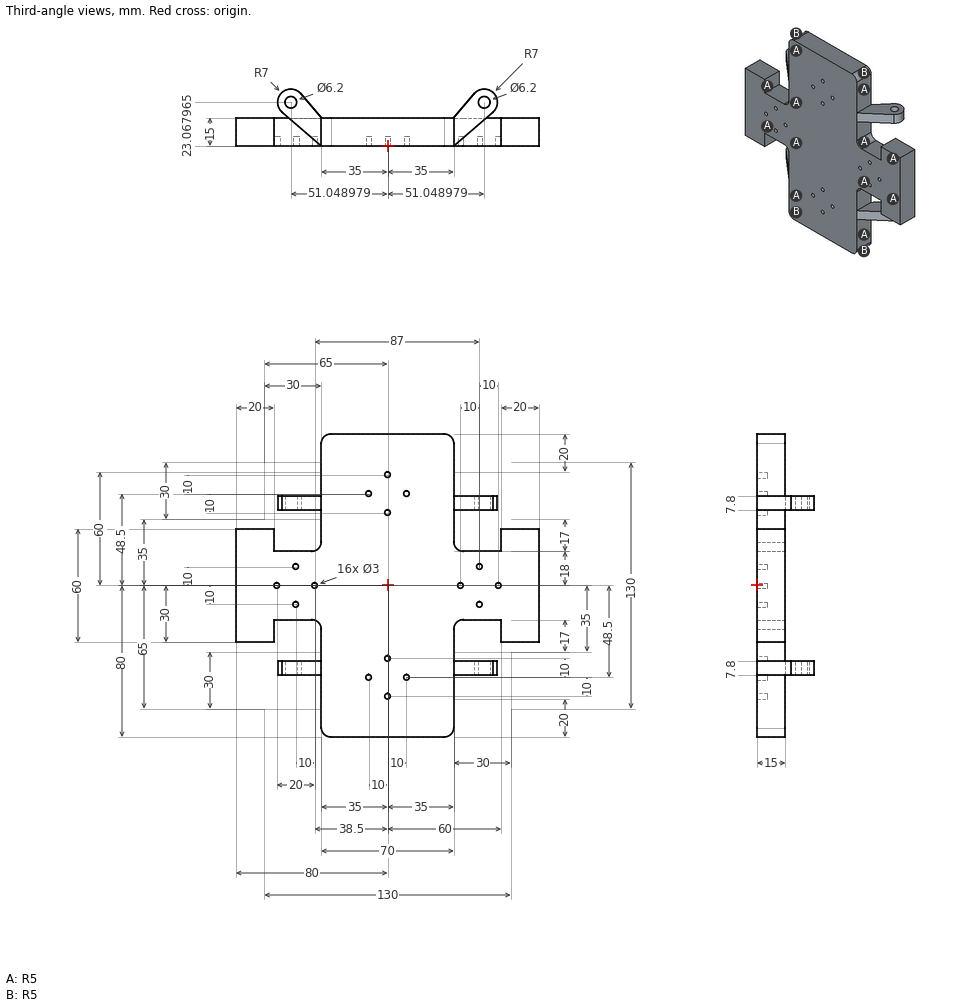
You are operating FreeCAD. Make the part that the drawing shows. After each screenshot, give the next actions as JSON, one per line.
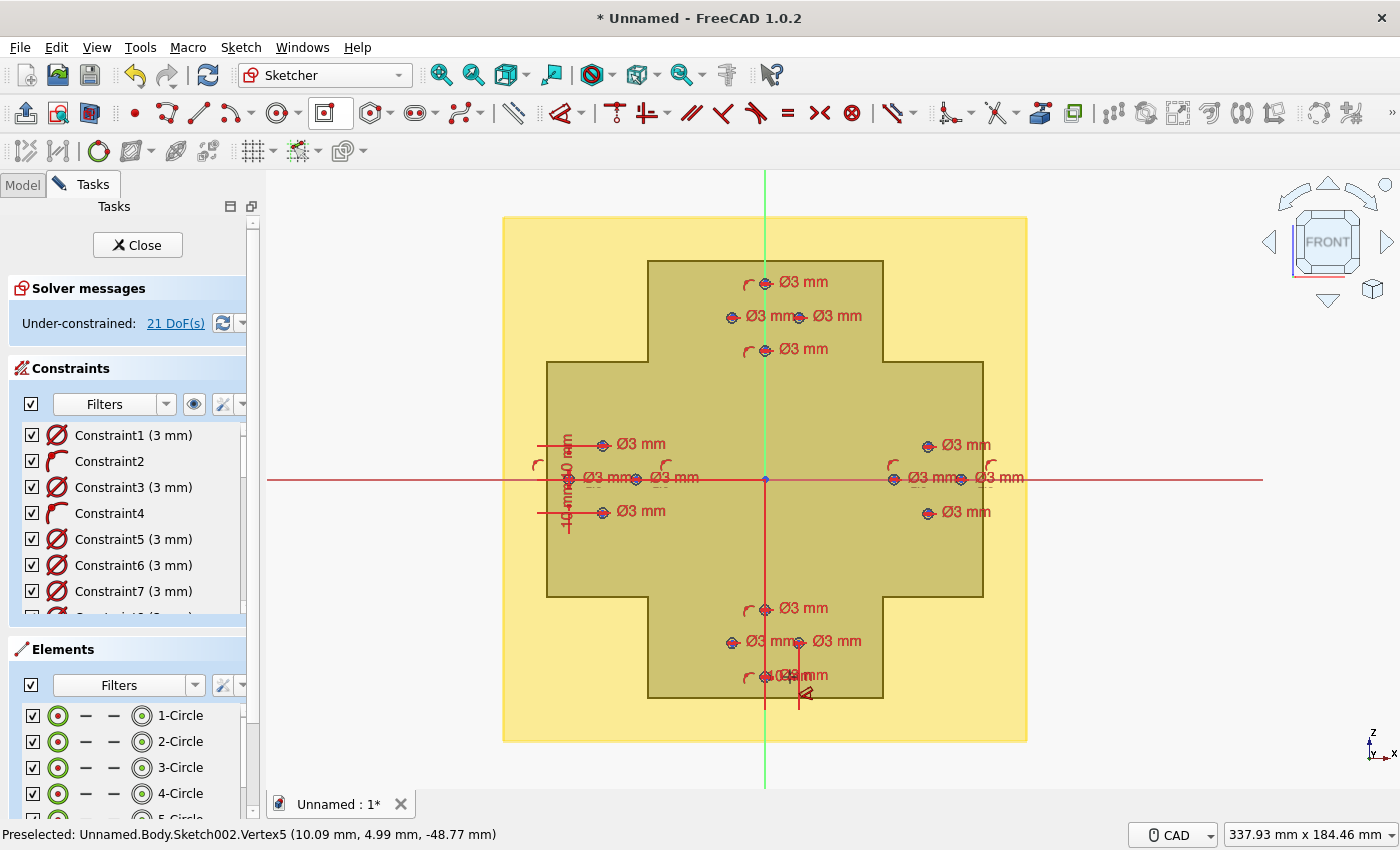
{"action": "left_click", "coordinate": [732, 643]}
{"action": "left_click", "coordinate": [749, 446]}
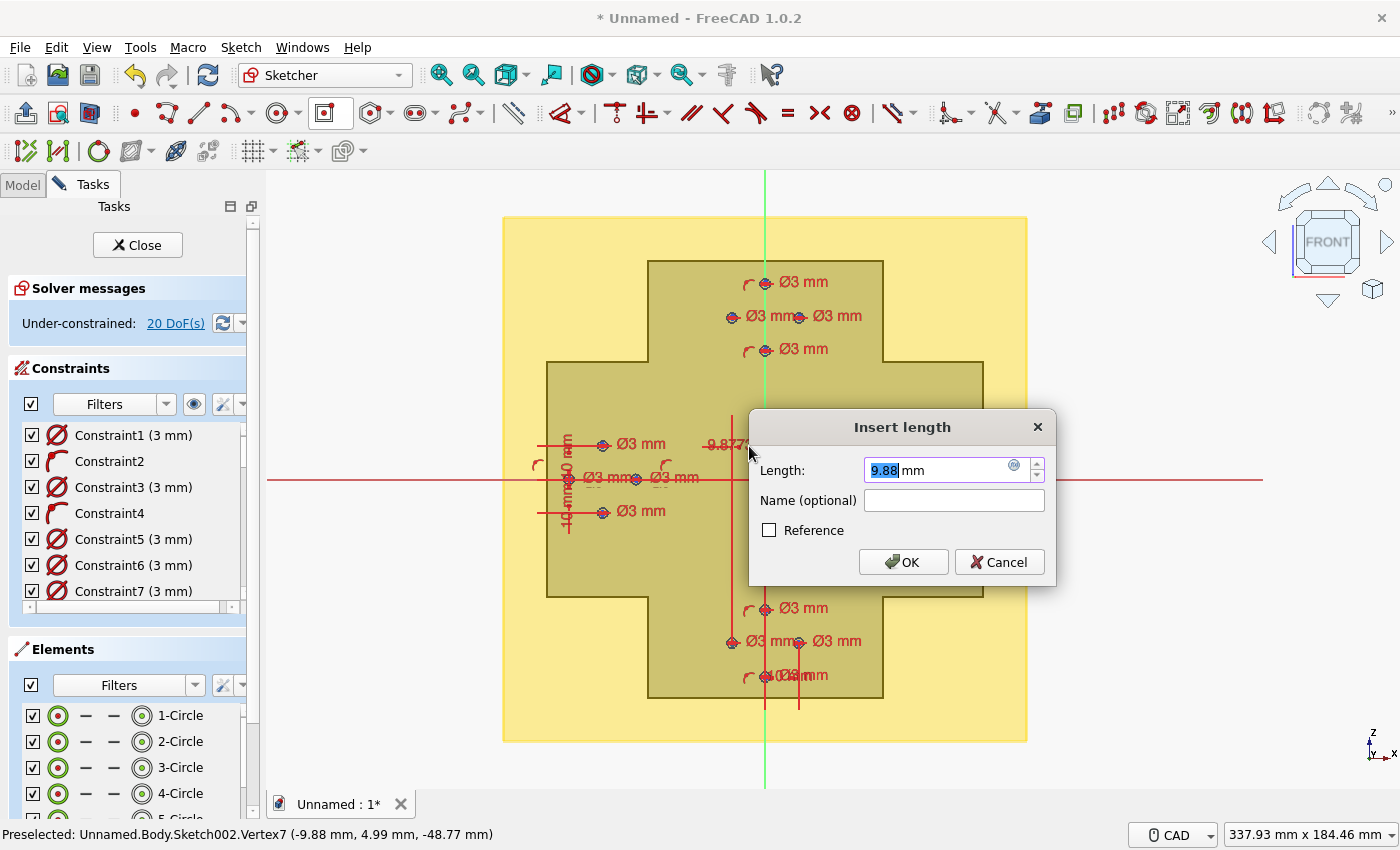
{"action": "type", "text": "10"}
{"action": "key", "text": "Return"}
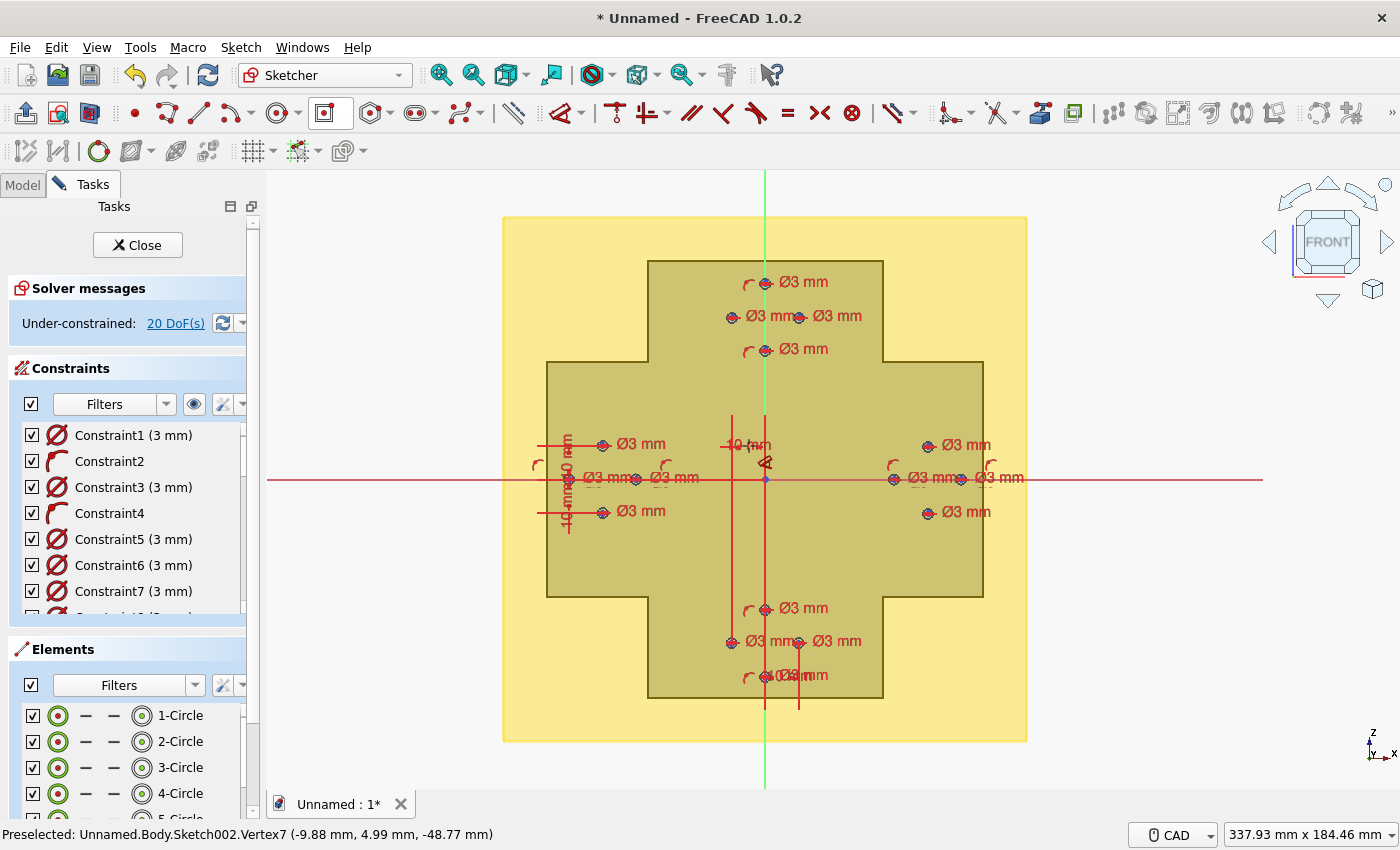
{"action": "left_click", "coordinate": [928, 447]}
{"action": "left_click", "coordinate": [962, 456]}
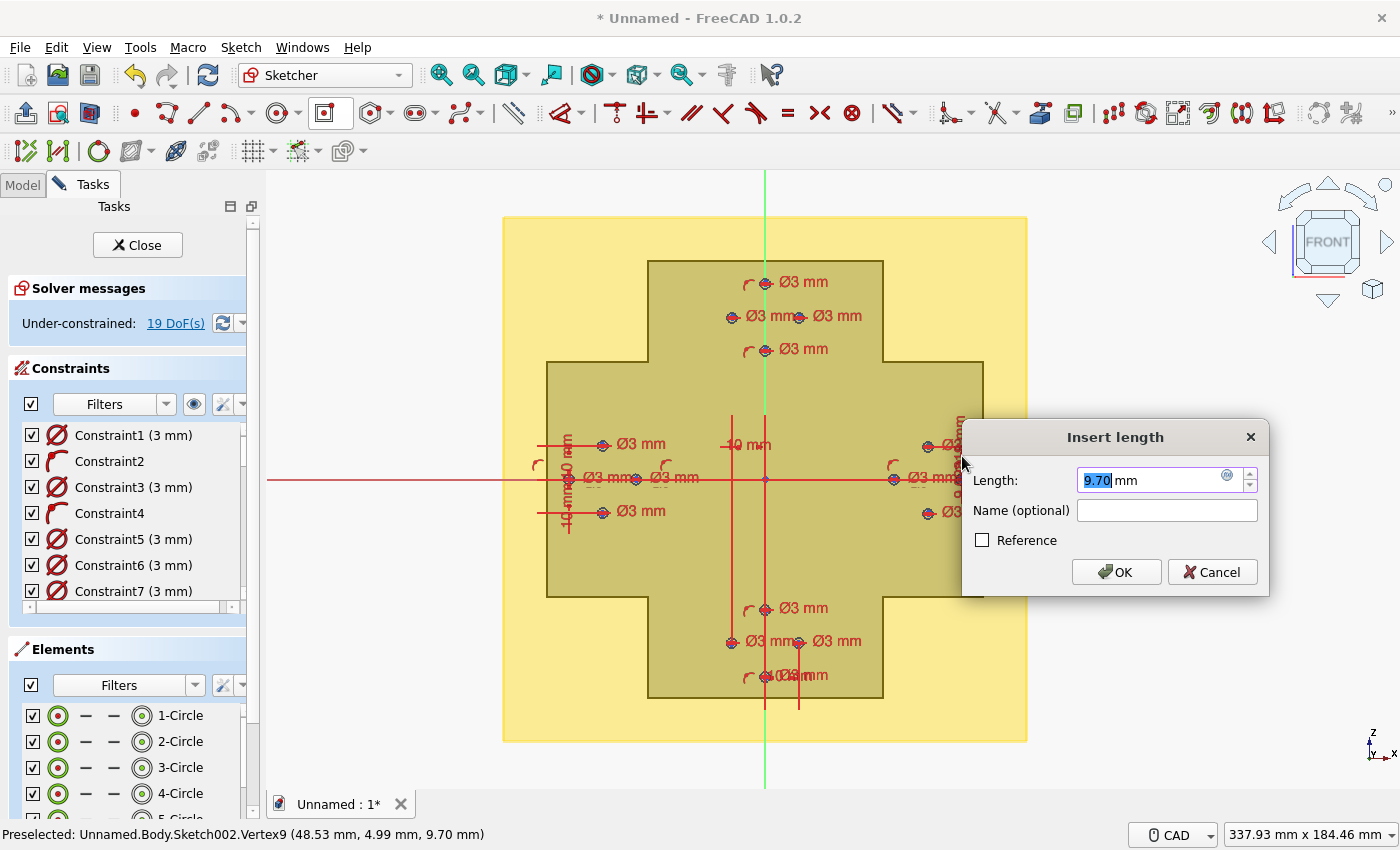
{"action": "type", "text": "10"}
{"action": "key", "text": "Return"}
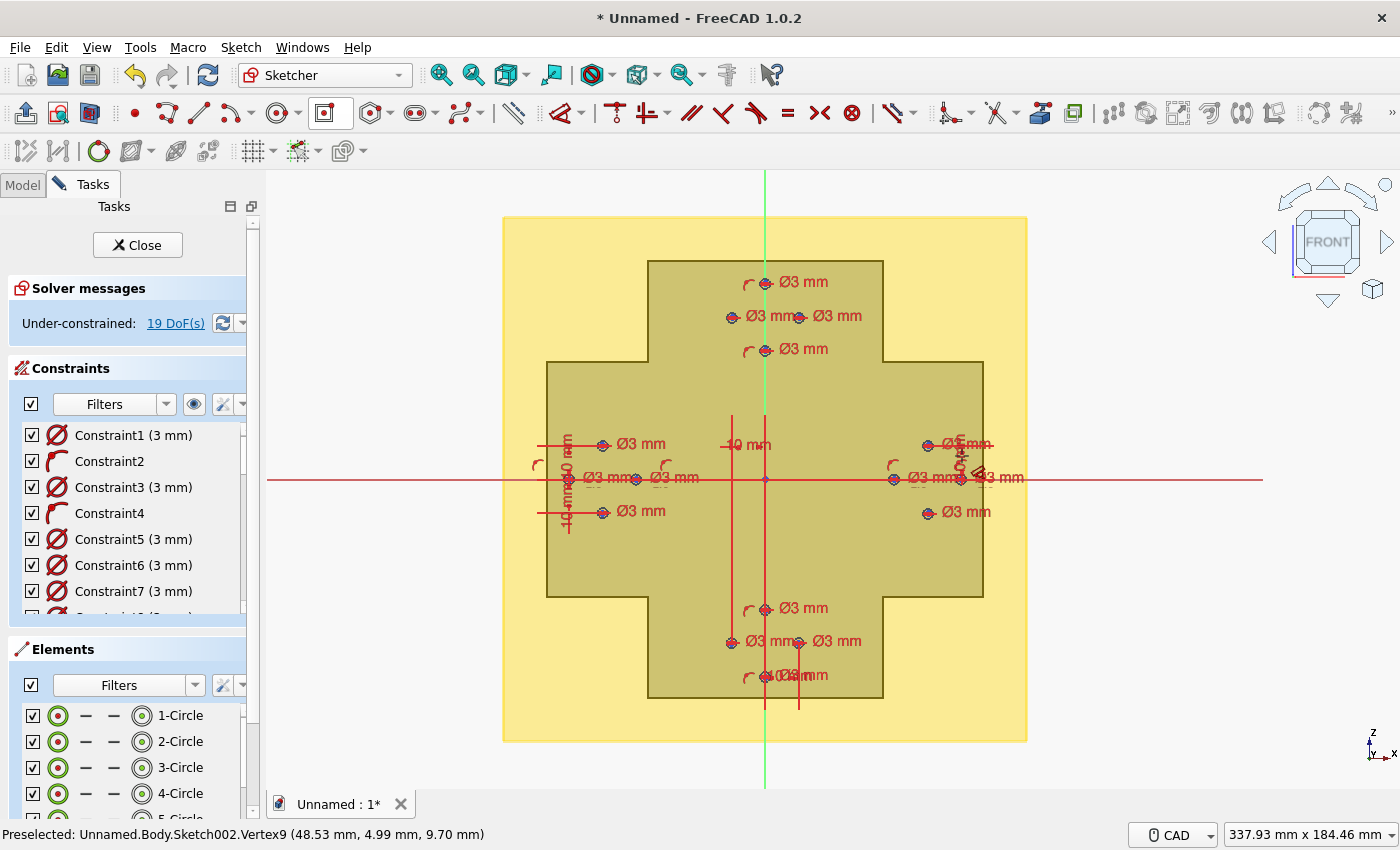
{"action": "left_click", "coordinate": [928, 514]}
{"action": "left_click", "coordinate": [962, 505]}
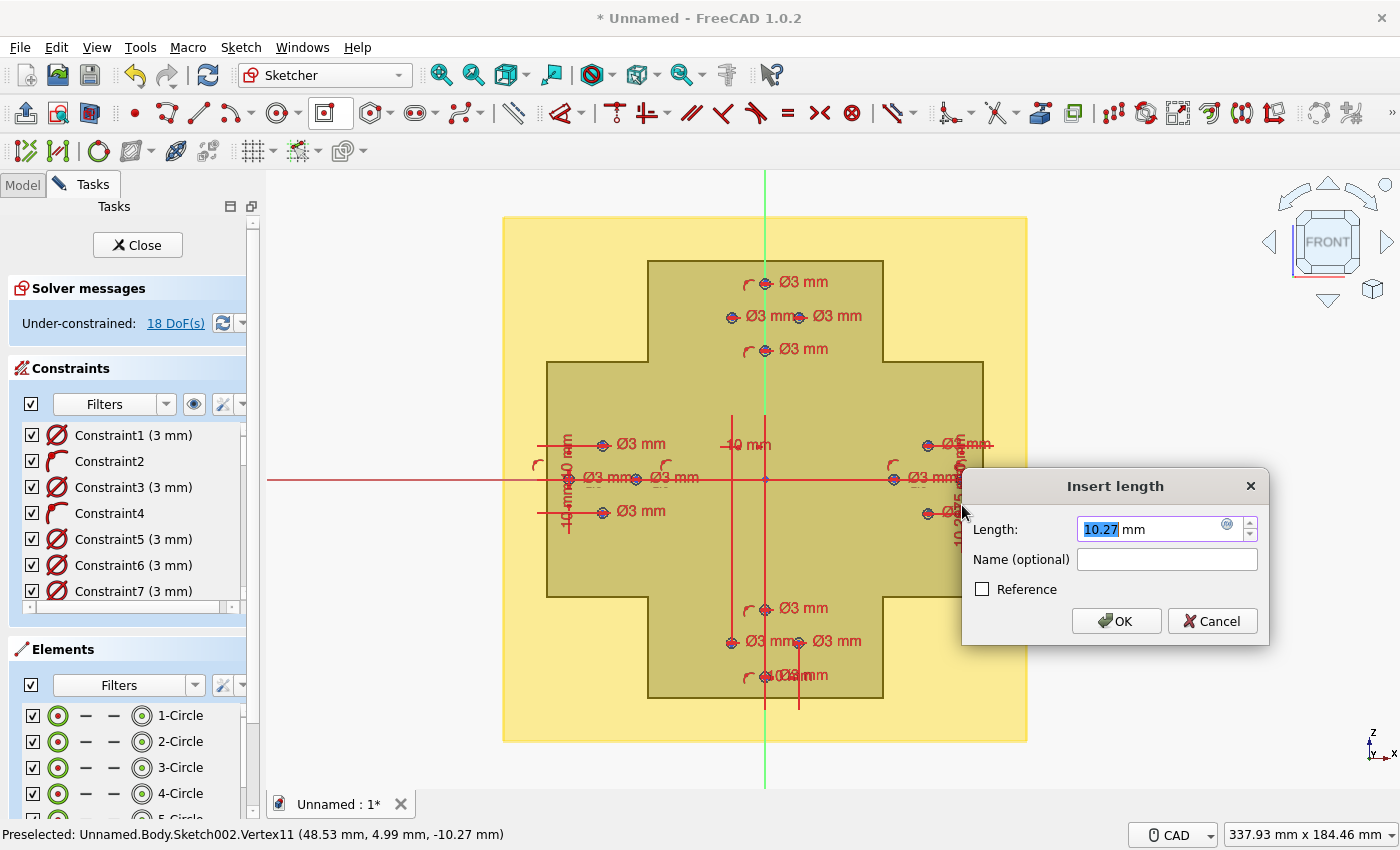
{"action": "type", "text": "10"}
{"action": "key", "text": "Return"}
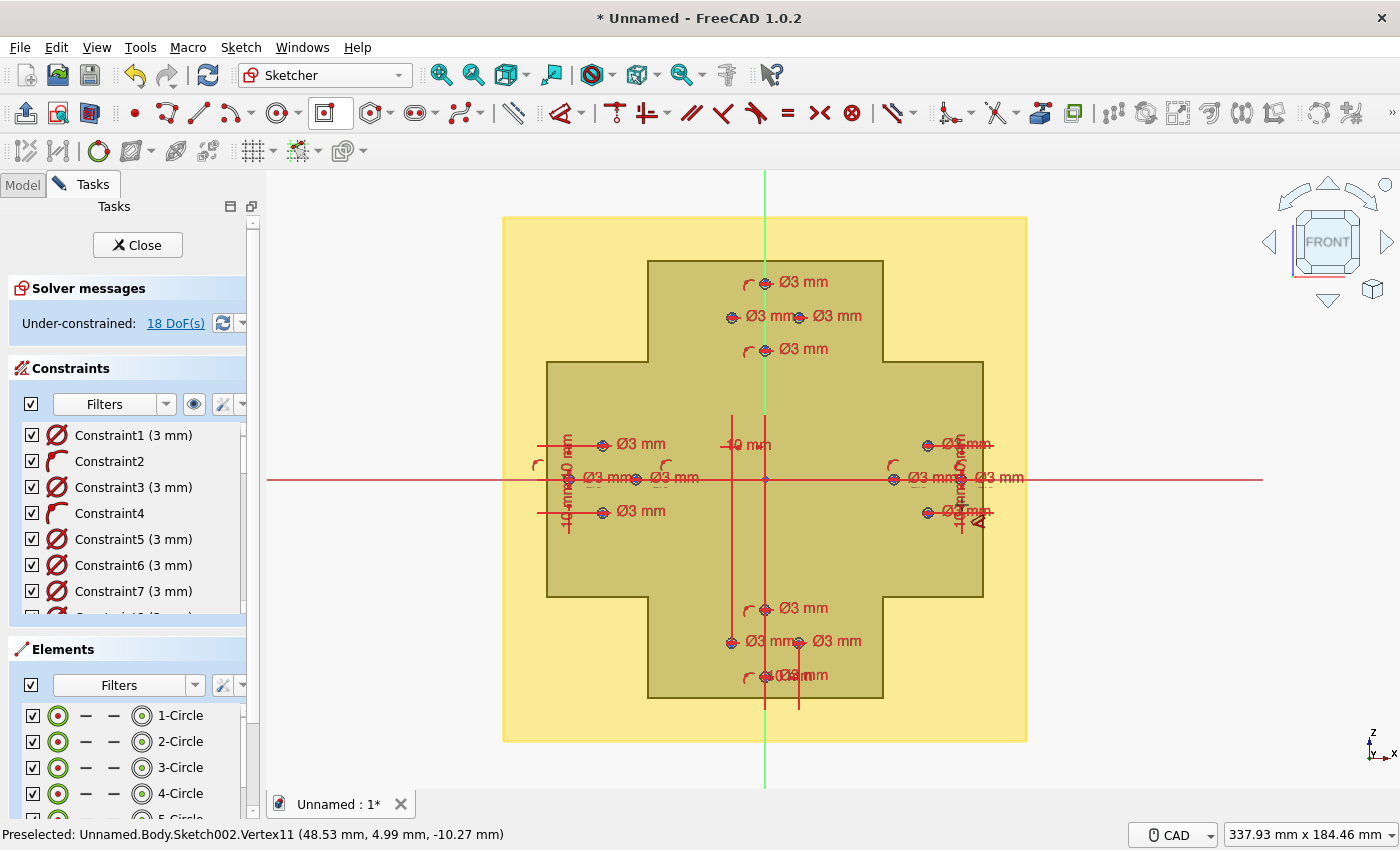
{"action": "left_click", "coordinate": [732, 318]}
{"action": "left_click", "coordinate": [741, 284]}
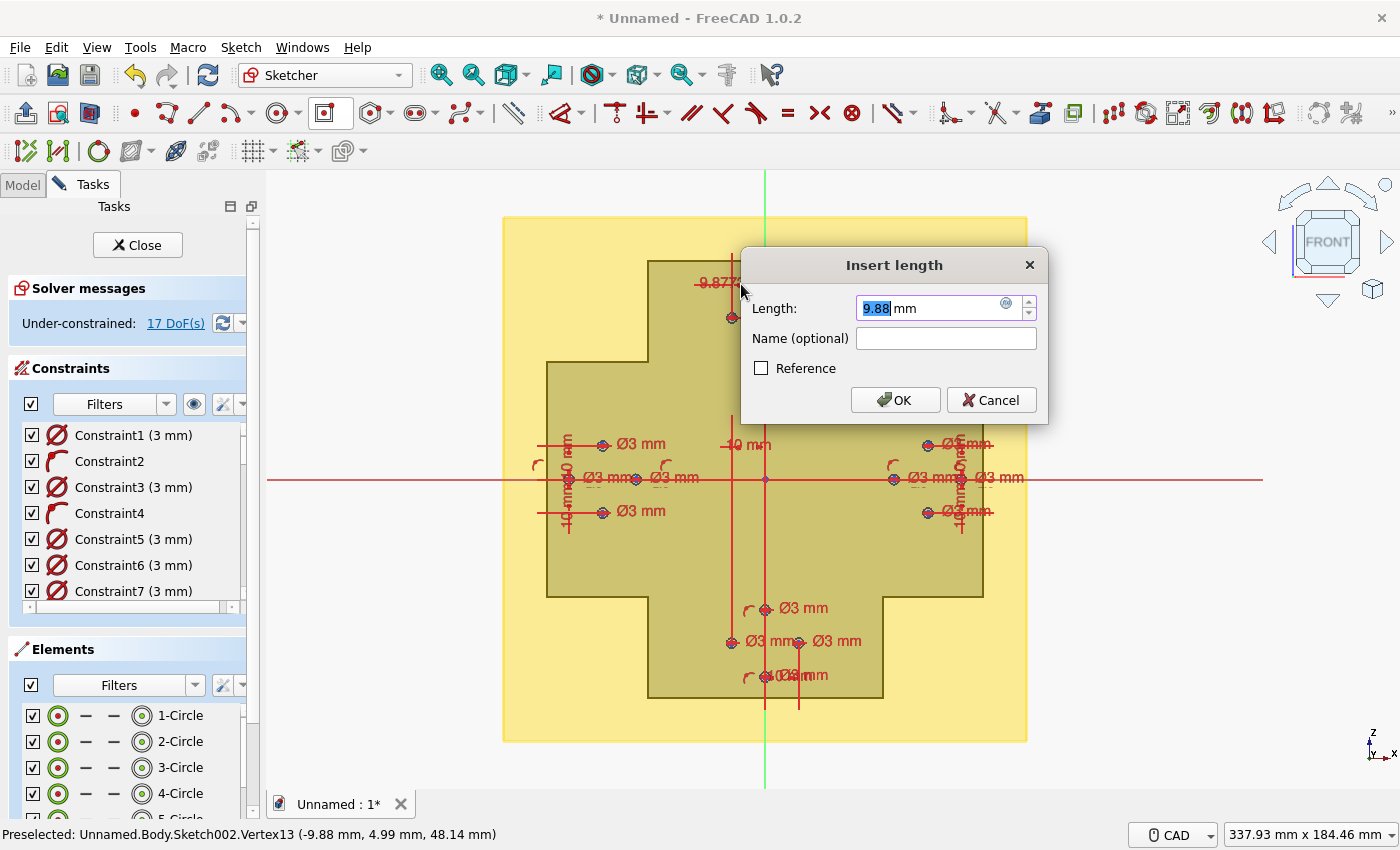
{"action": "type", "text": "10"}
{"action": "key", "text": "Return"}